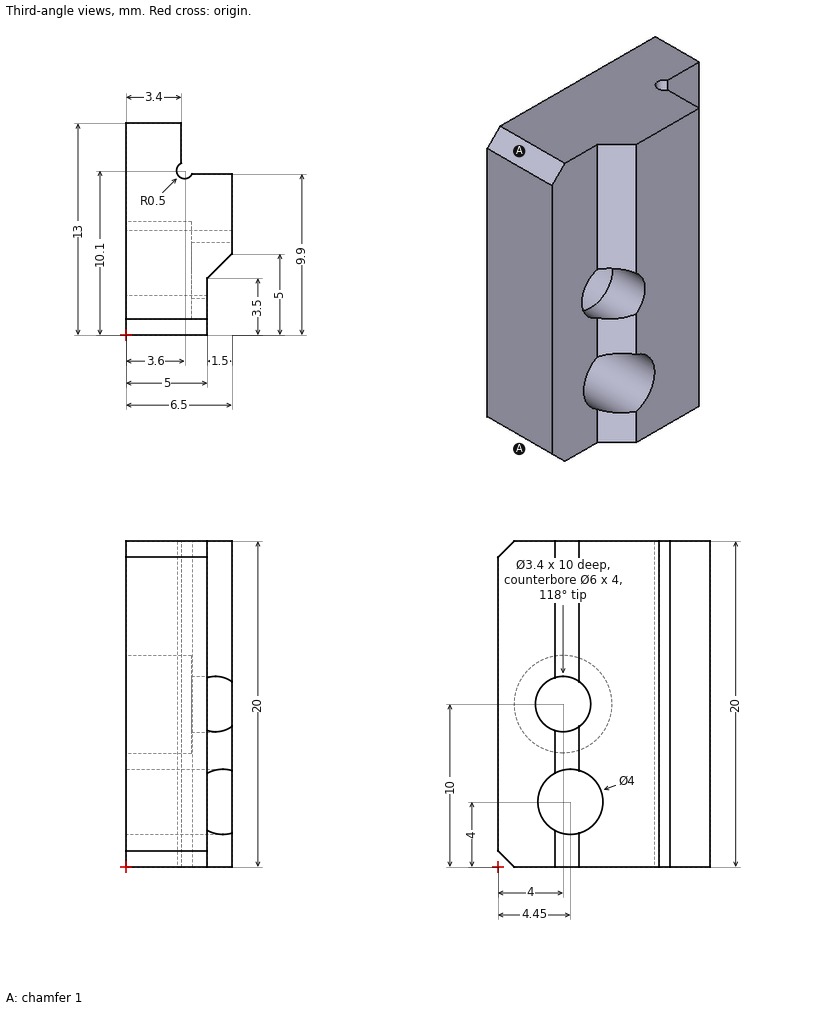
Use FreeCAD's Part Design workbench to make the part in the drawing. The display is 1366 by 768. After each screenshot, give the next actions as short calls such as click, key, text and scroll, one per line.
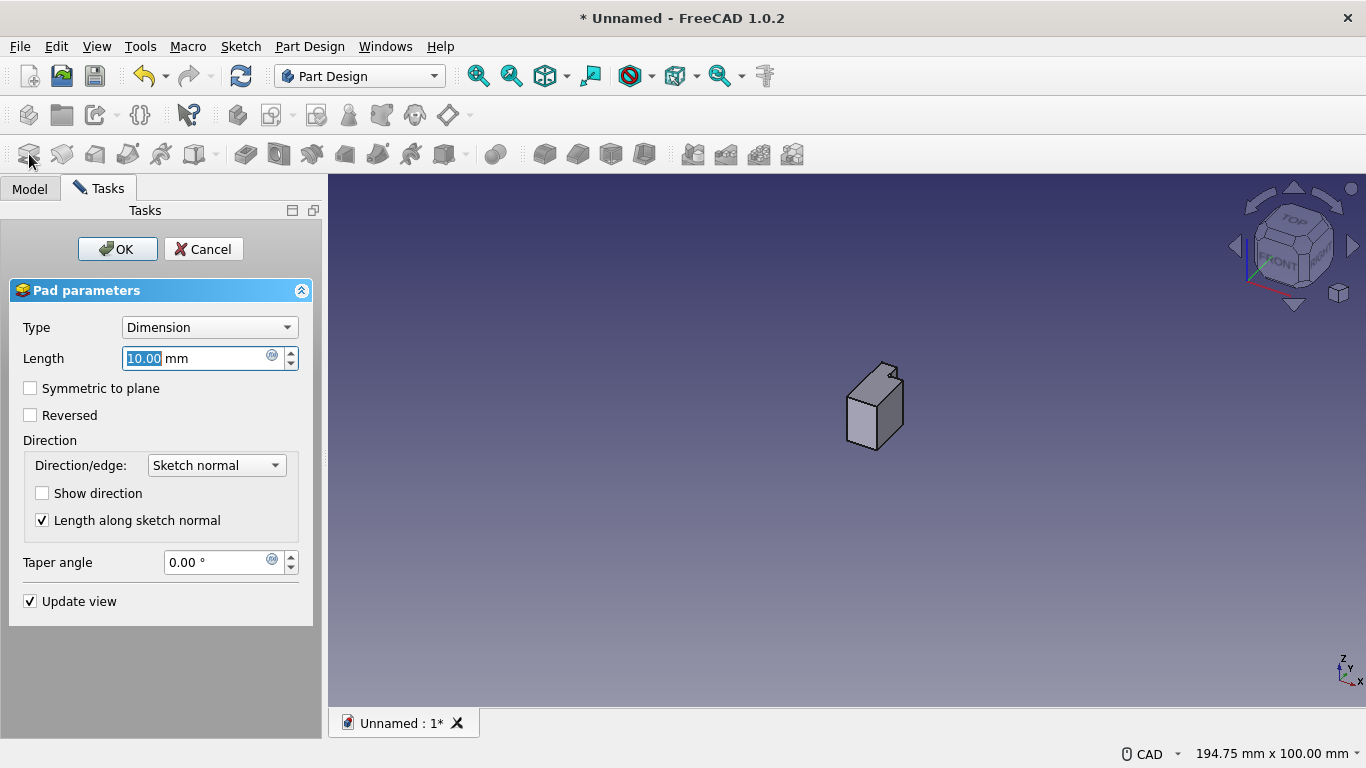
text(20)
key(Tab)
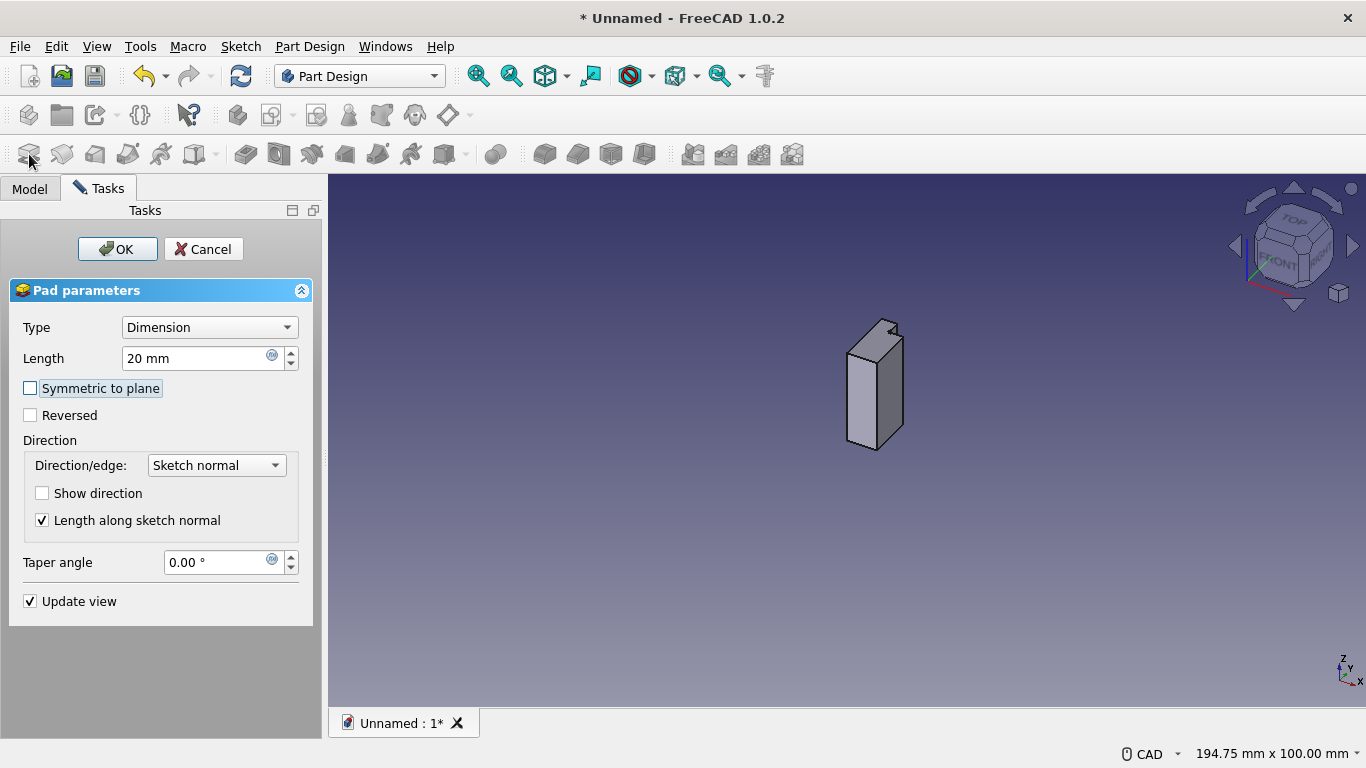
click(118, 249)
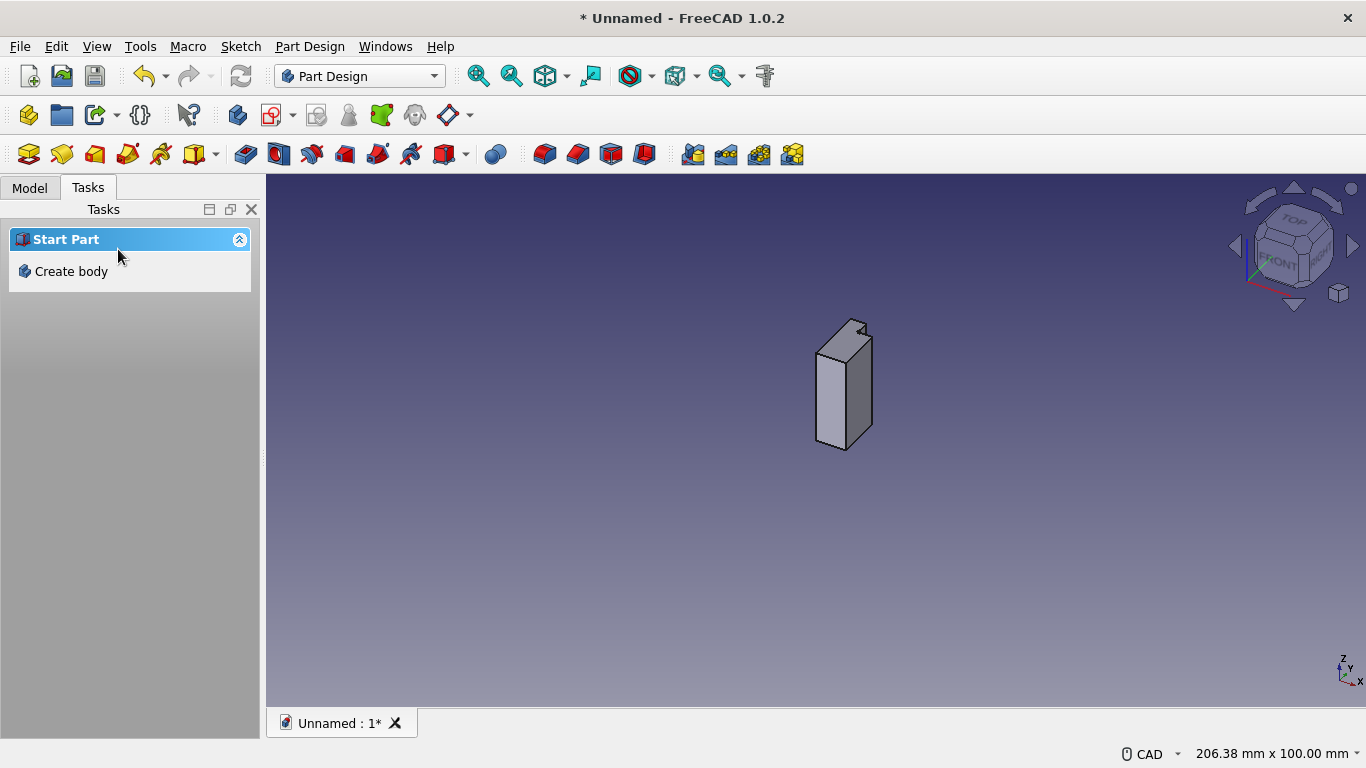
click(479, 76)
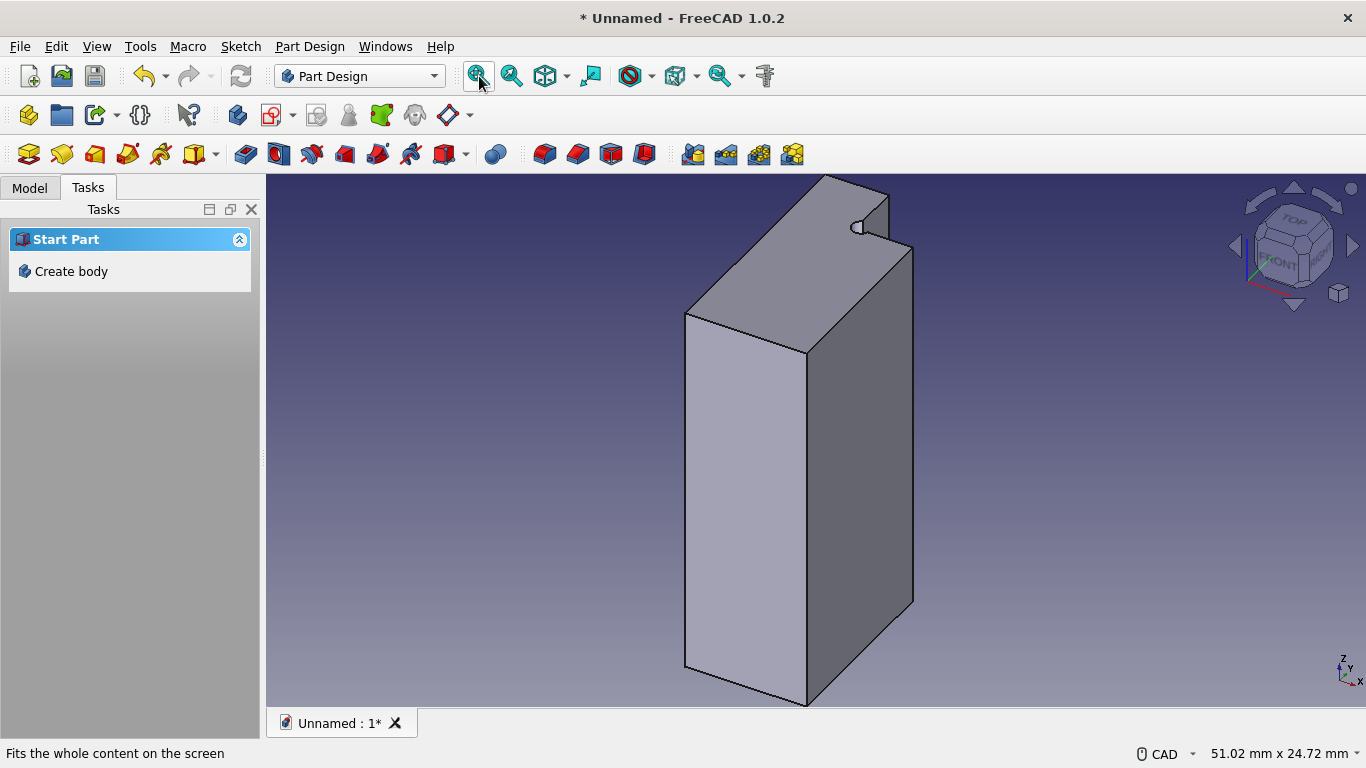
click(796, 283)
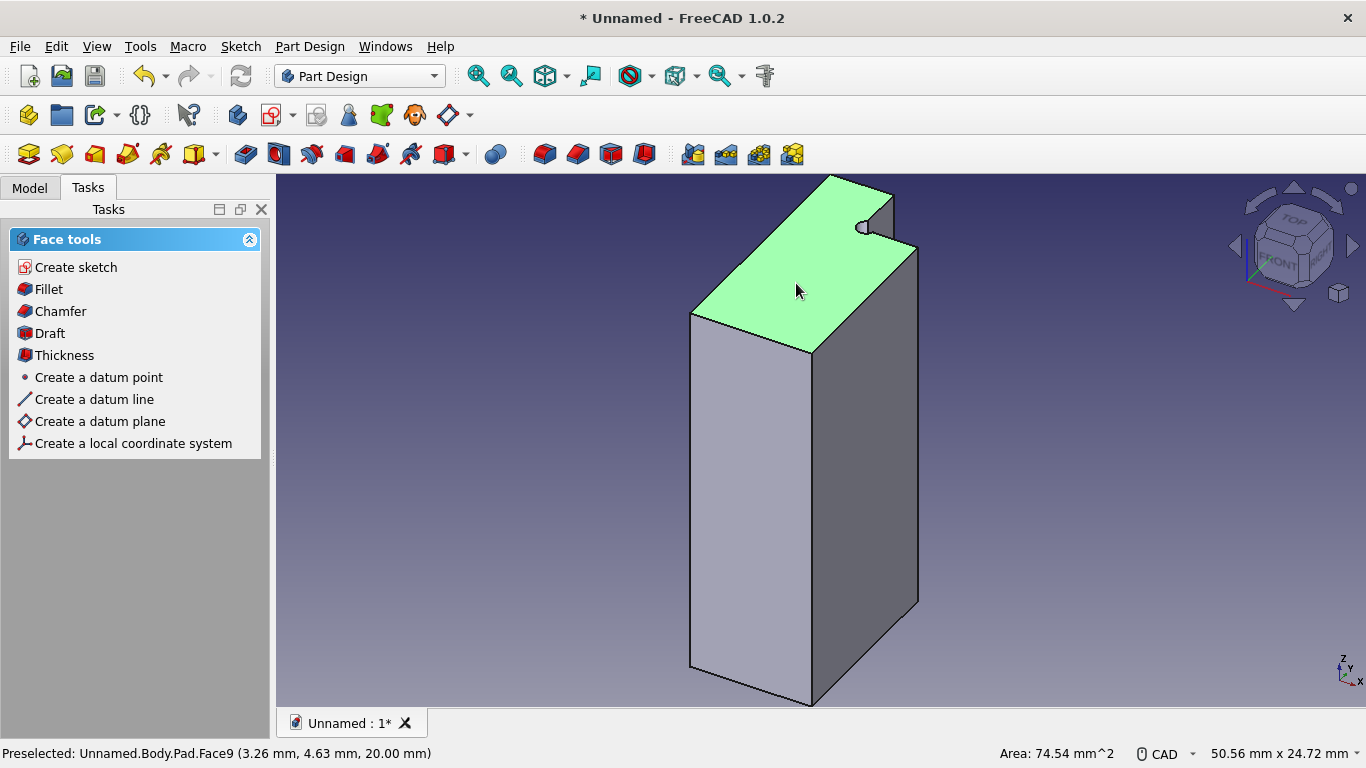
click(270, 116)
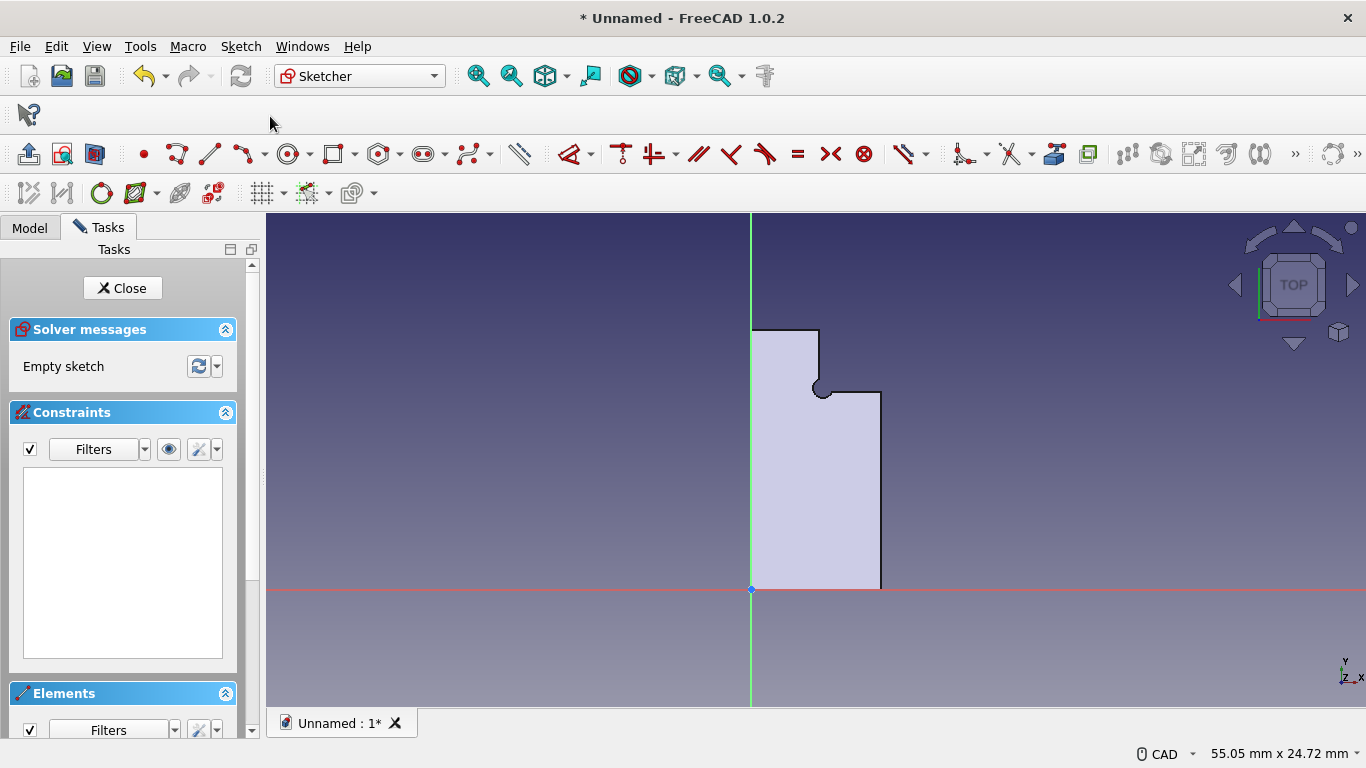
scroll(846, 574, up, 6)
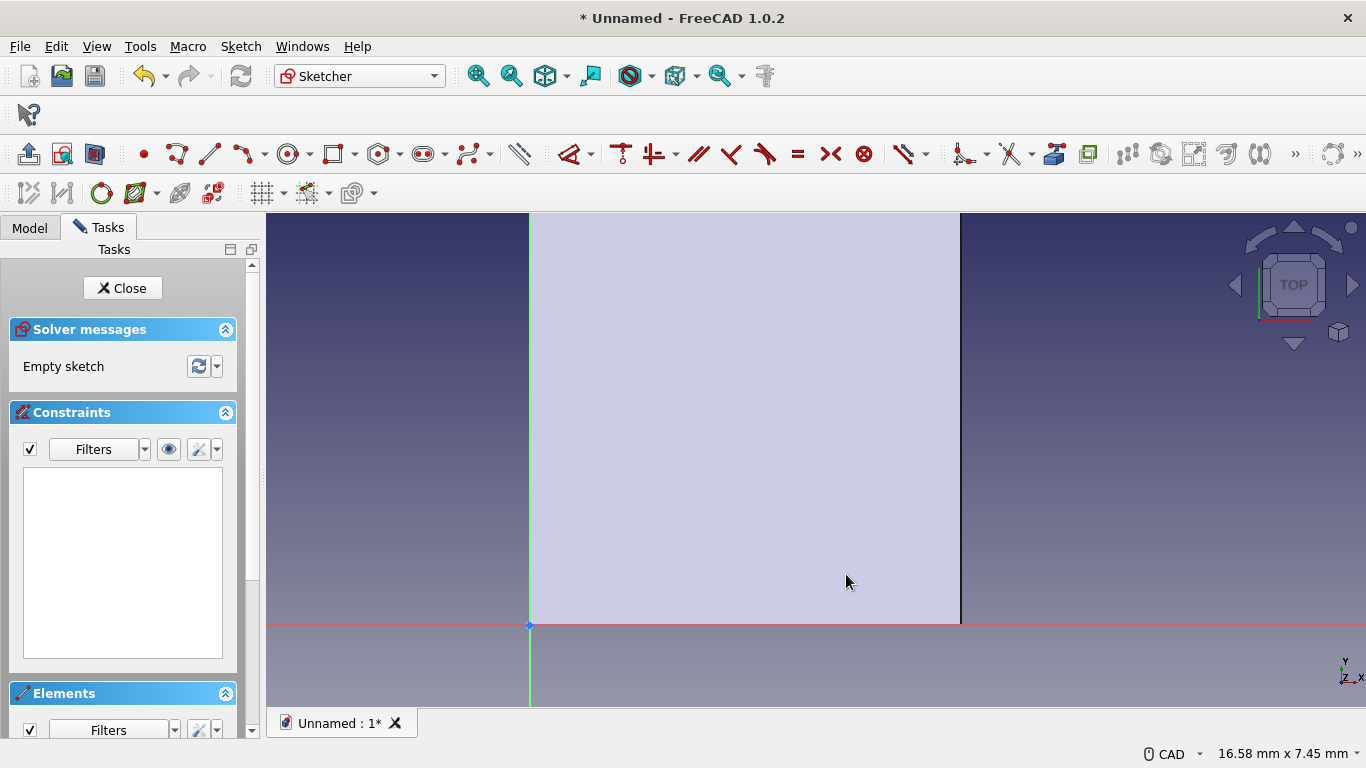
click(177, 154)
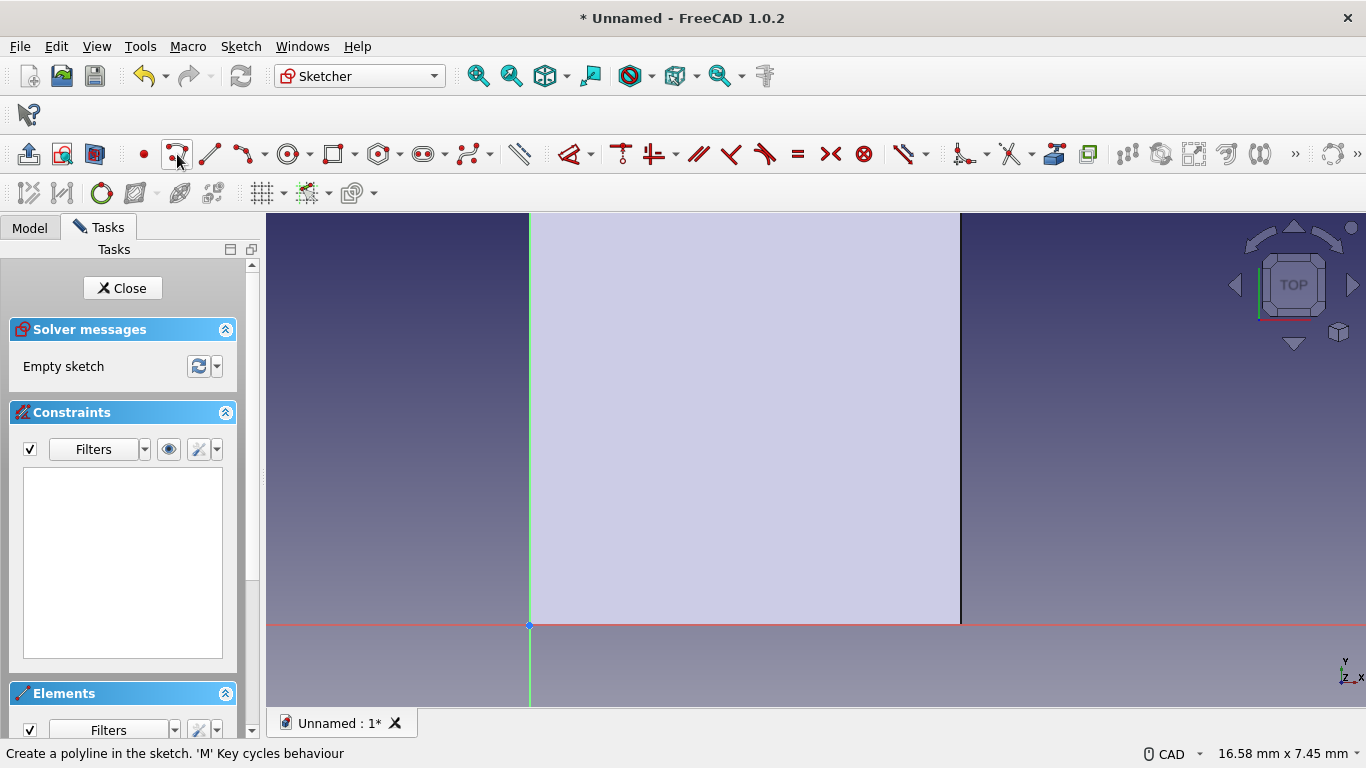
click(861, 625)
click(961, 616)
click(961, 293)
click(861, 393)
click(861, 625)
key(Escape)
key(Escape)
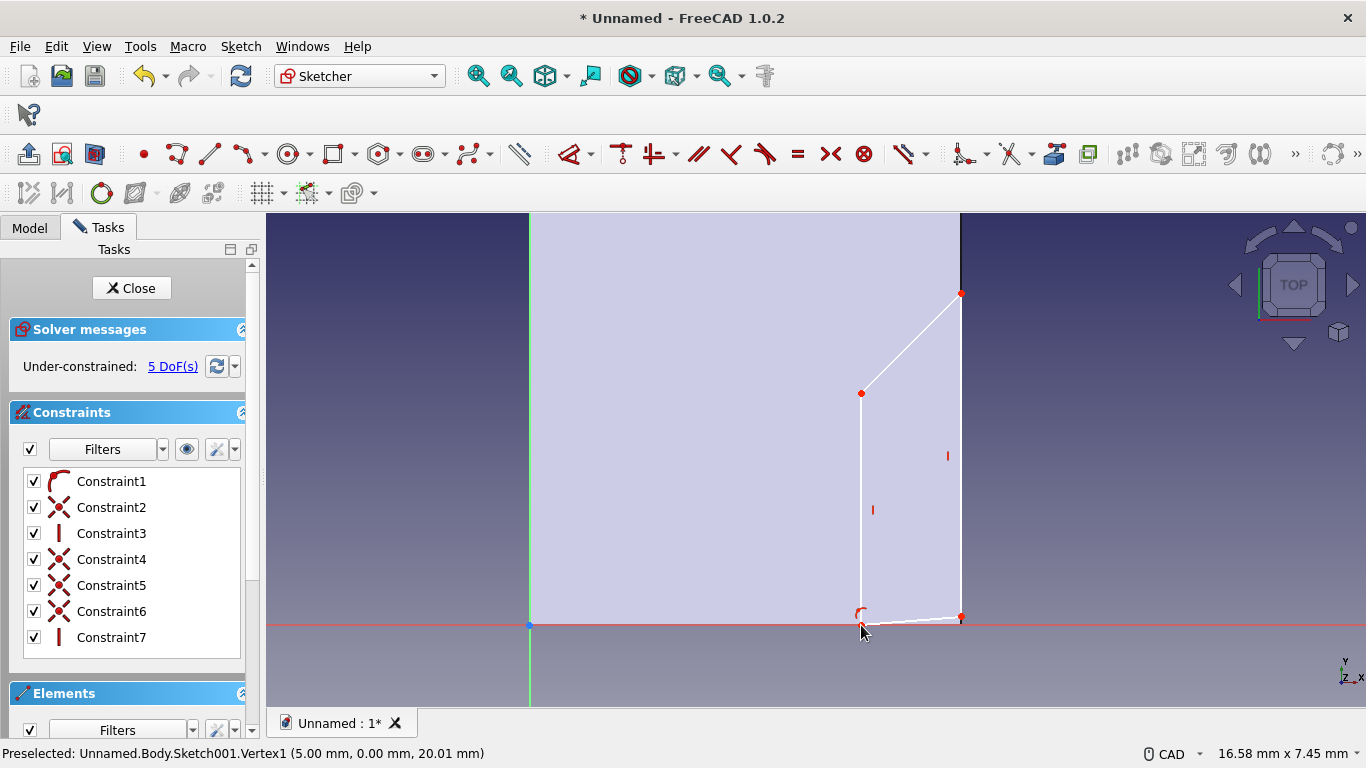
click(891, 623)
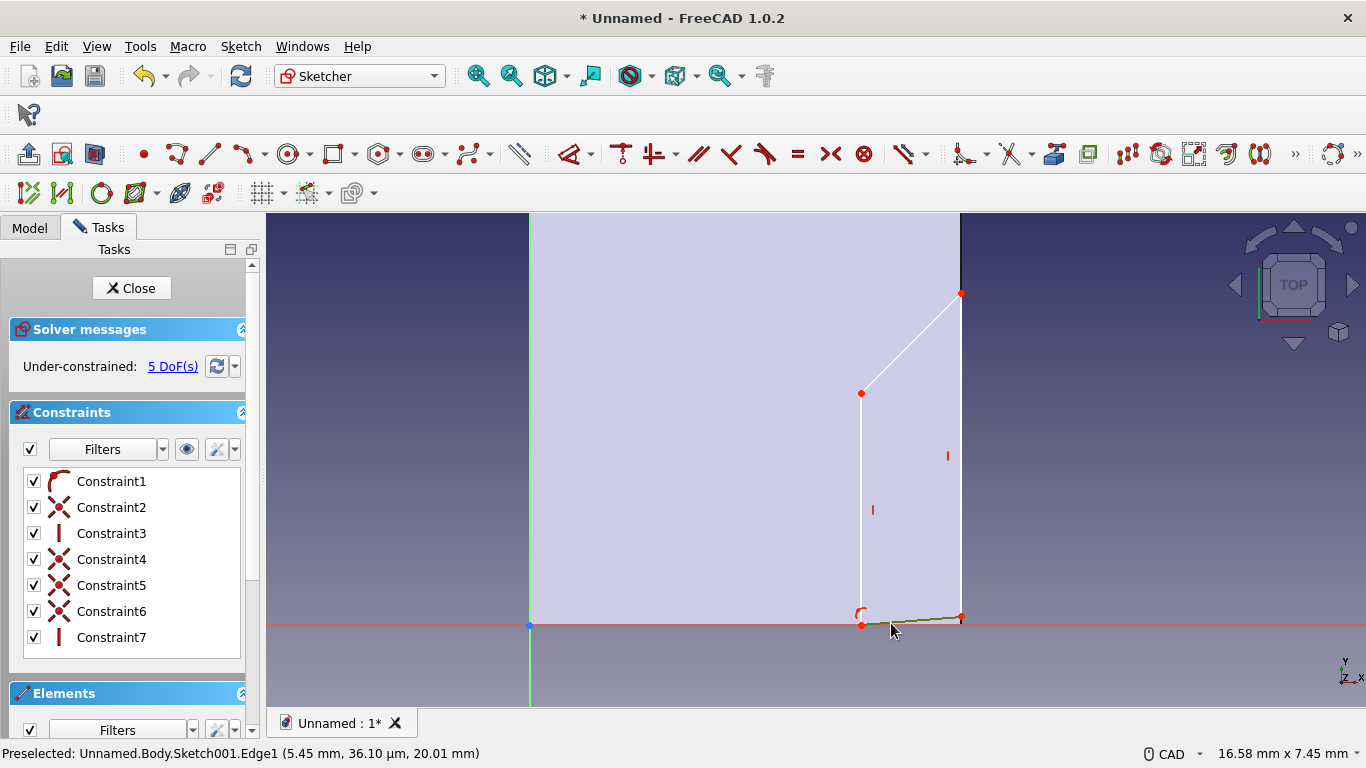
click(676, 154)